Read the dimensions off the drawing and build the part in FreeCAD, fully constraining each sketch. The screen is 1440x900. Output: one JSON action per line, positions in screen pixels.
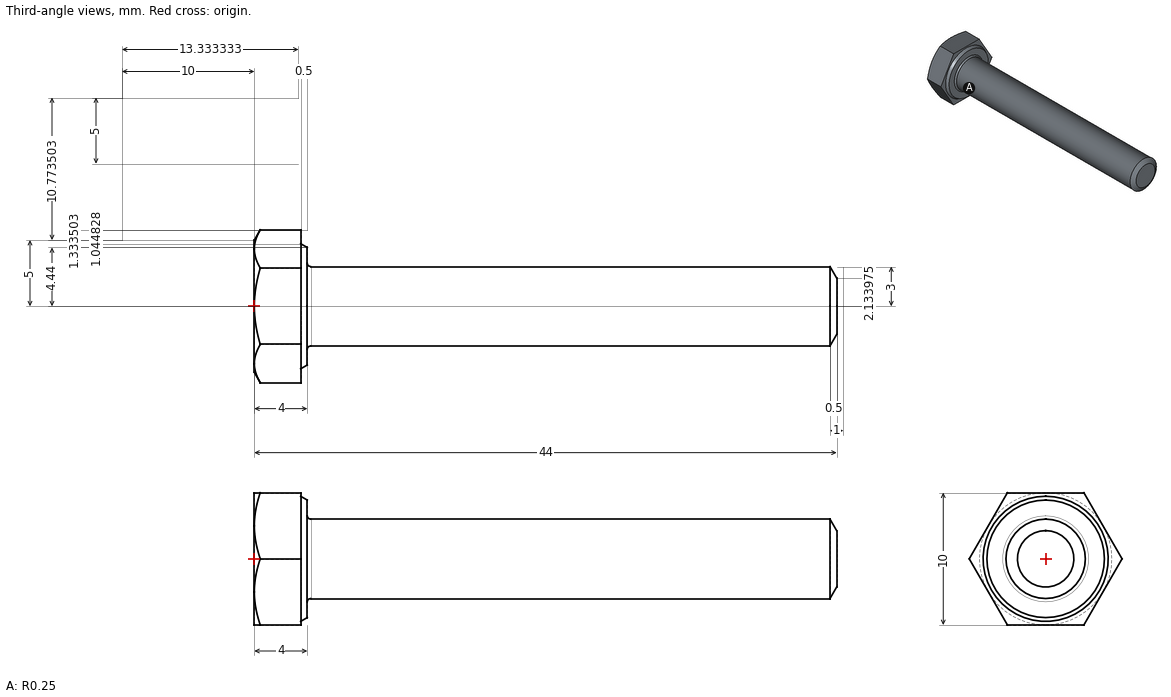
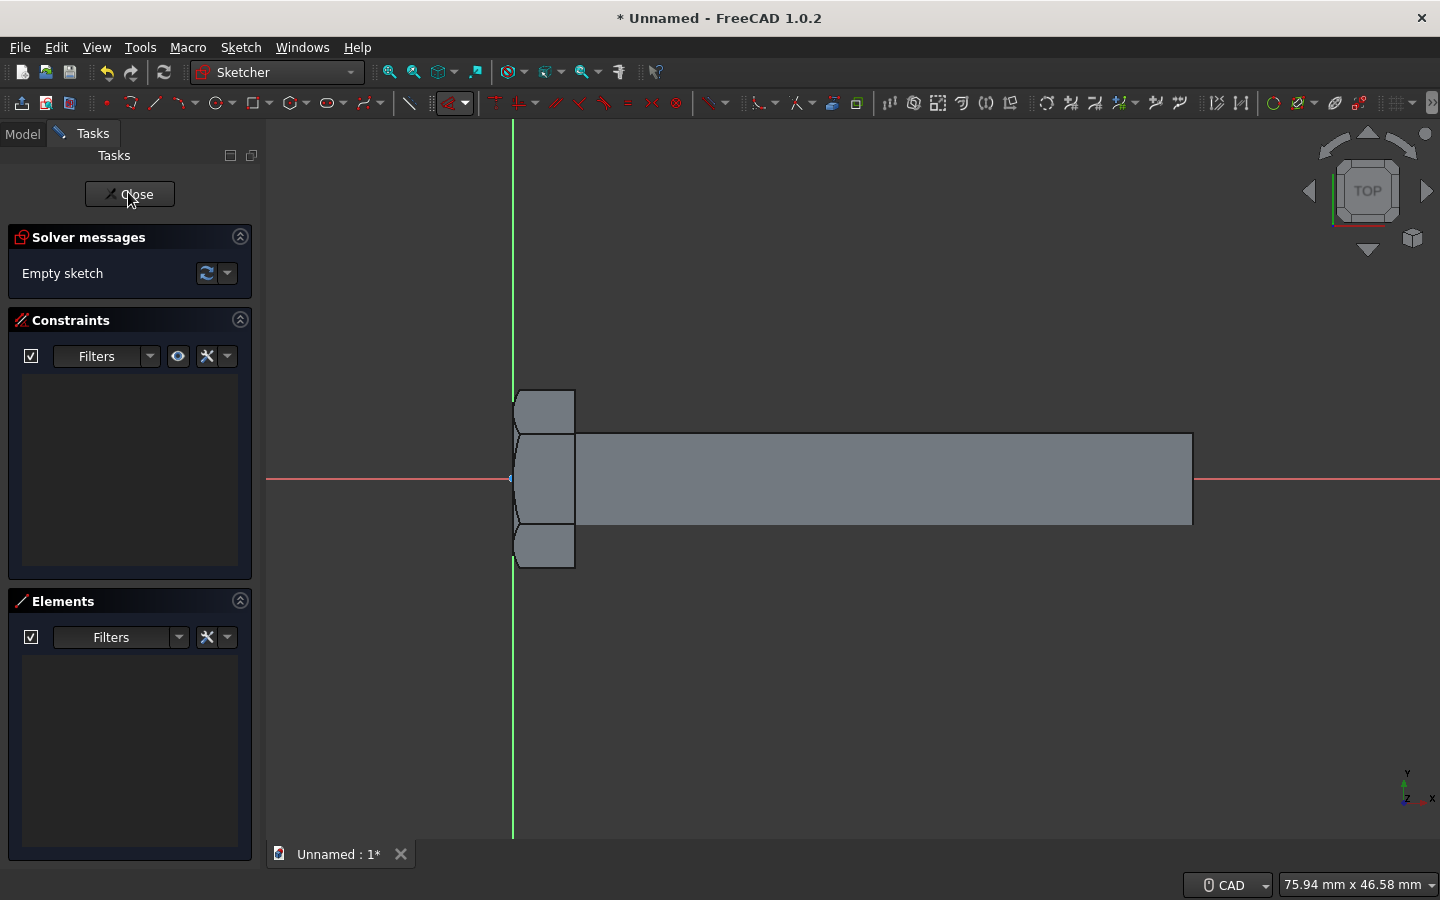
{"action": "left_click", "coordinate": [70, 104]}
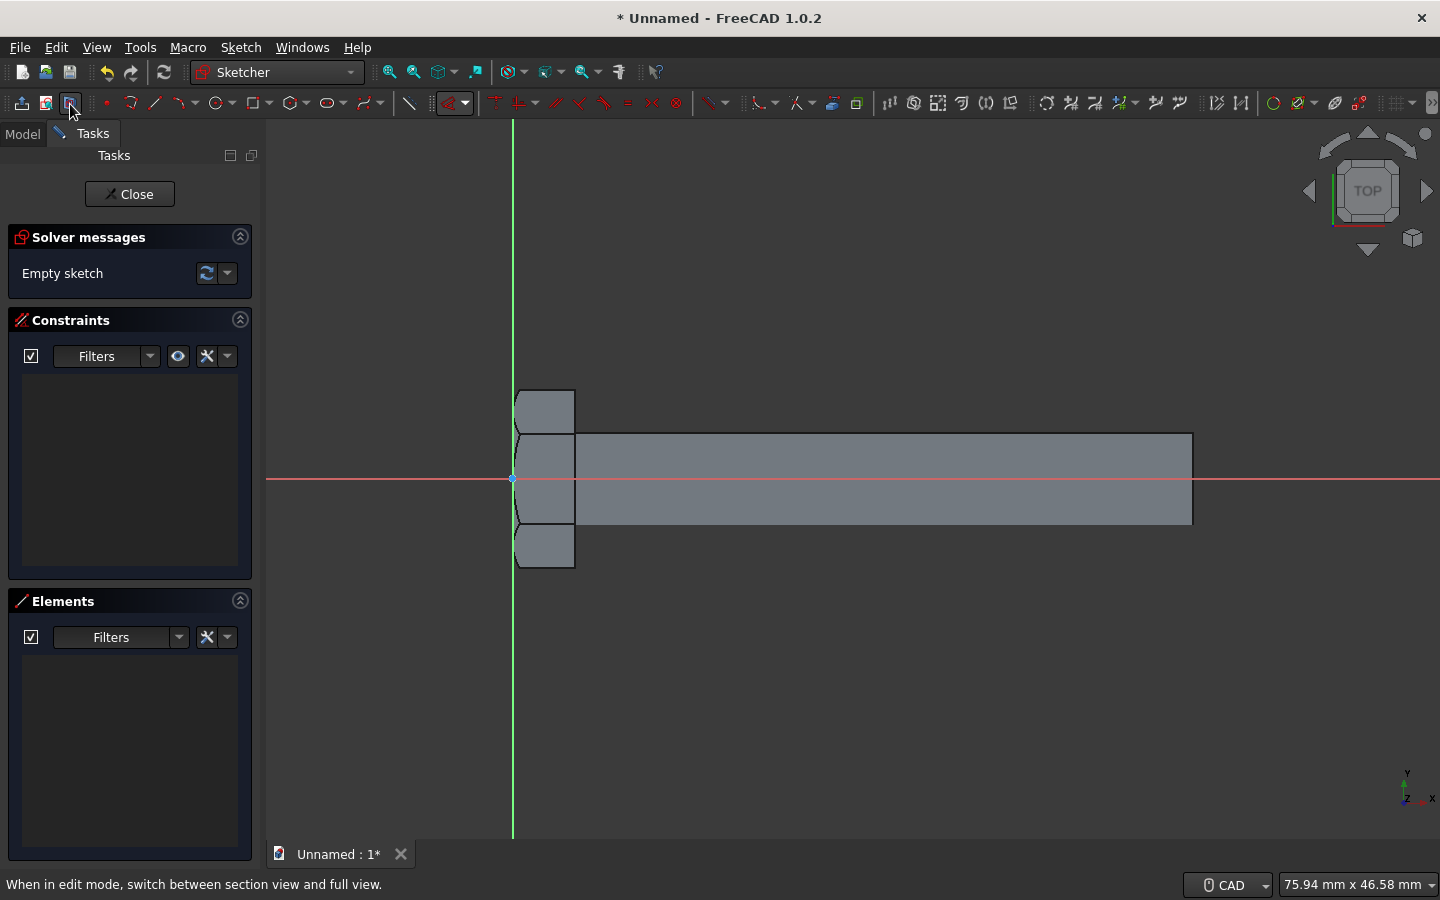
{"action": "scroll", "coordinate": [560, 396], "scroll_direction": "up", "scroll_amount": 15}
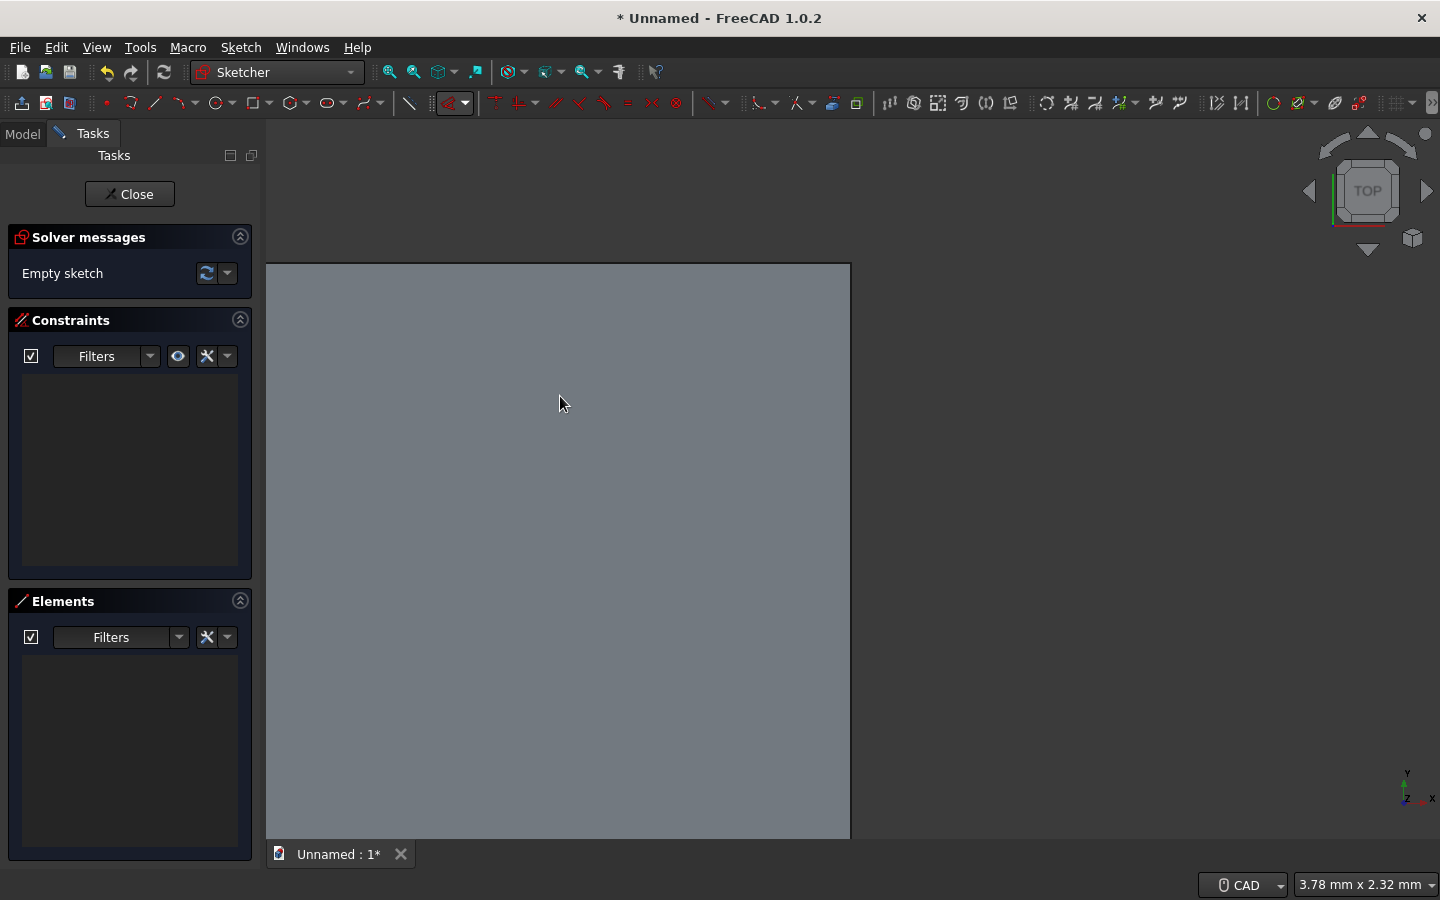
{"action": "left_click", "coordinate": [132, 104]}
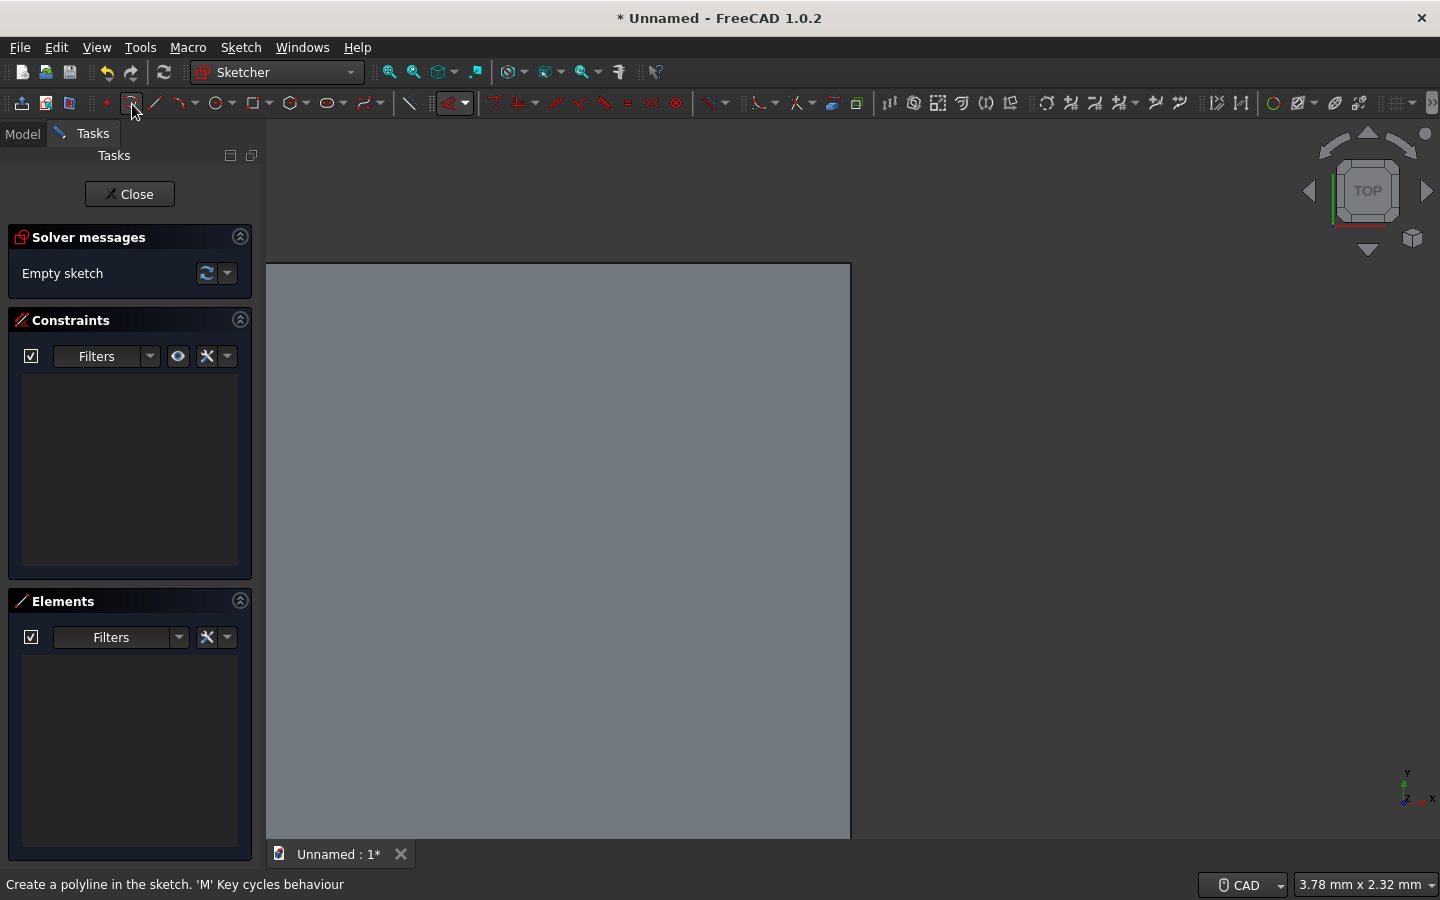
{"action": "left_click", "coordinate": [696, 588]}
{"action": "left_click", "coordinate": [851, 677]}
{"action": "left_click", "coordinate": [851, 263]}
{"action": "left_click", "coordinate": [696, 263]}
{"action": "left_click", "coordinate": [696, 589]}
{"action": "key", "text": "Escape"}
{"action": "key", "text": "Escape"}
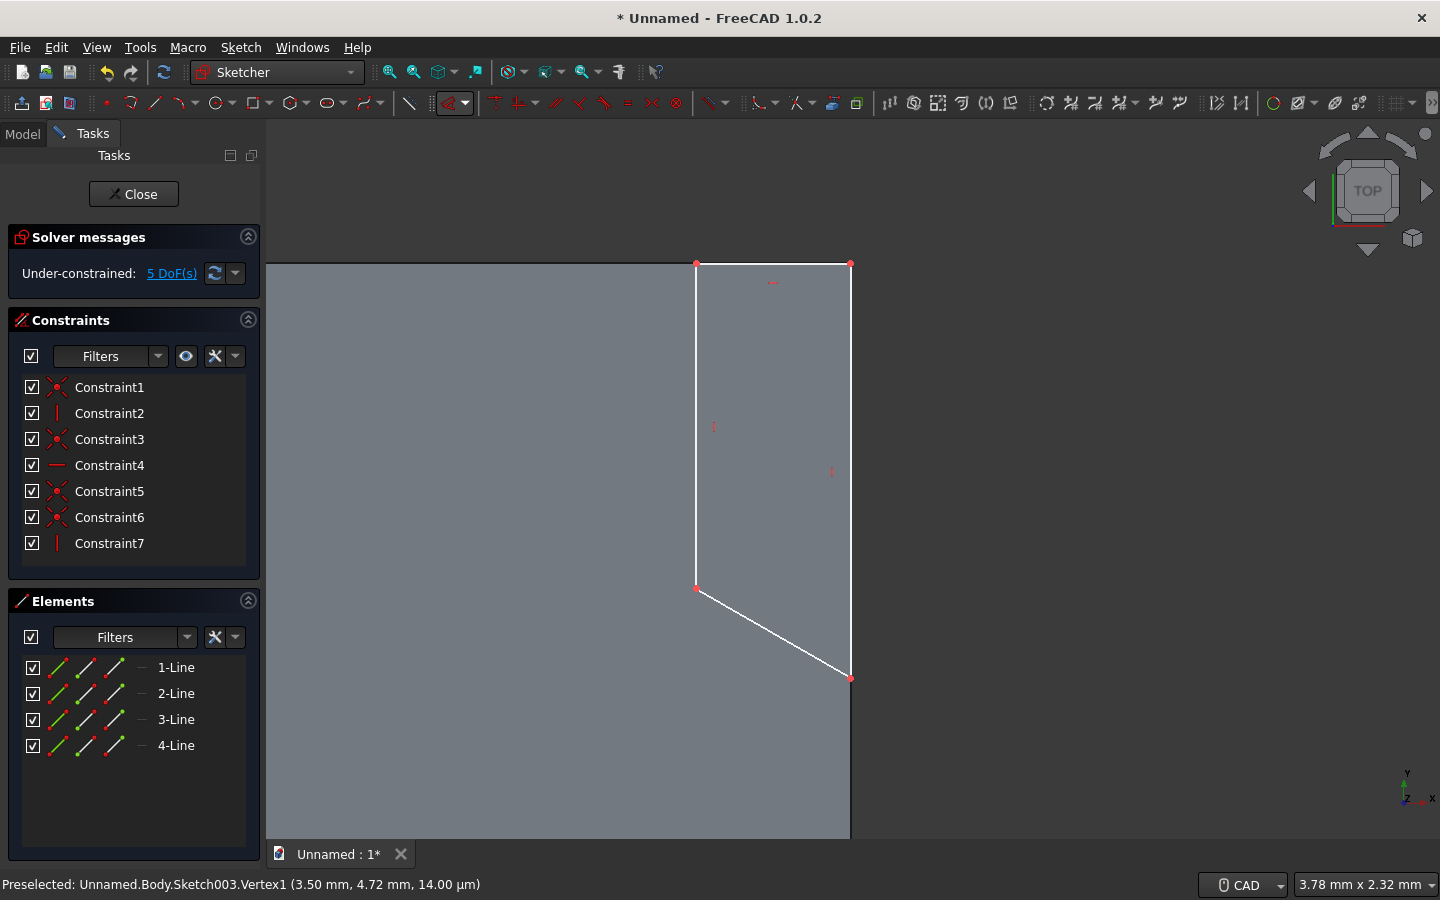
{"action": "left_click", "coordinate": [851, 678]}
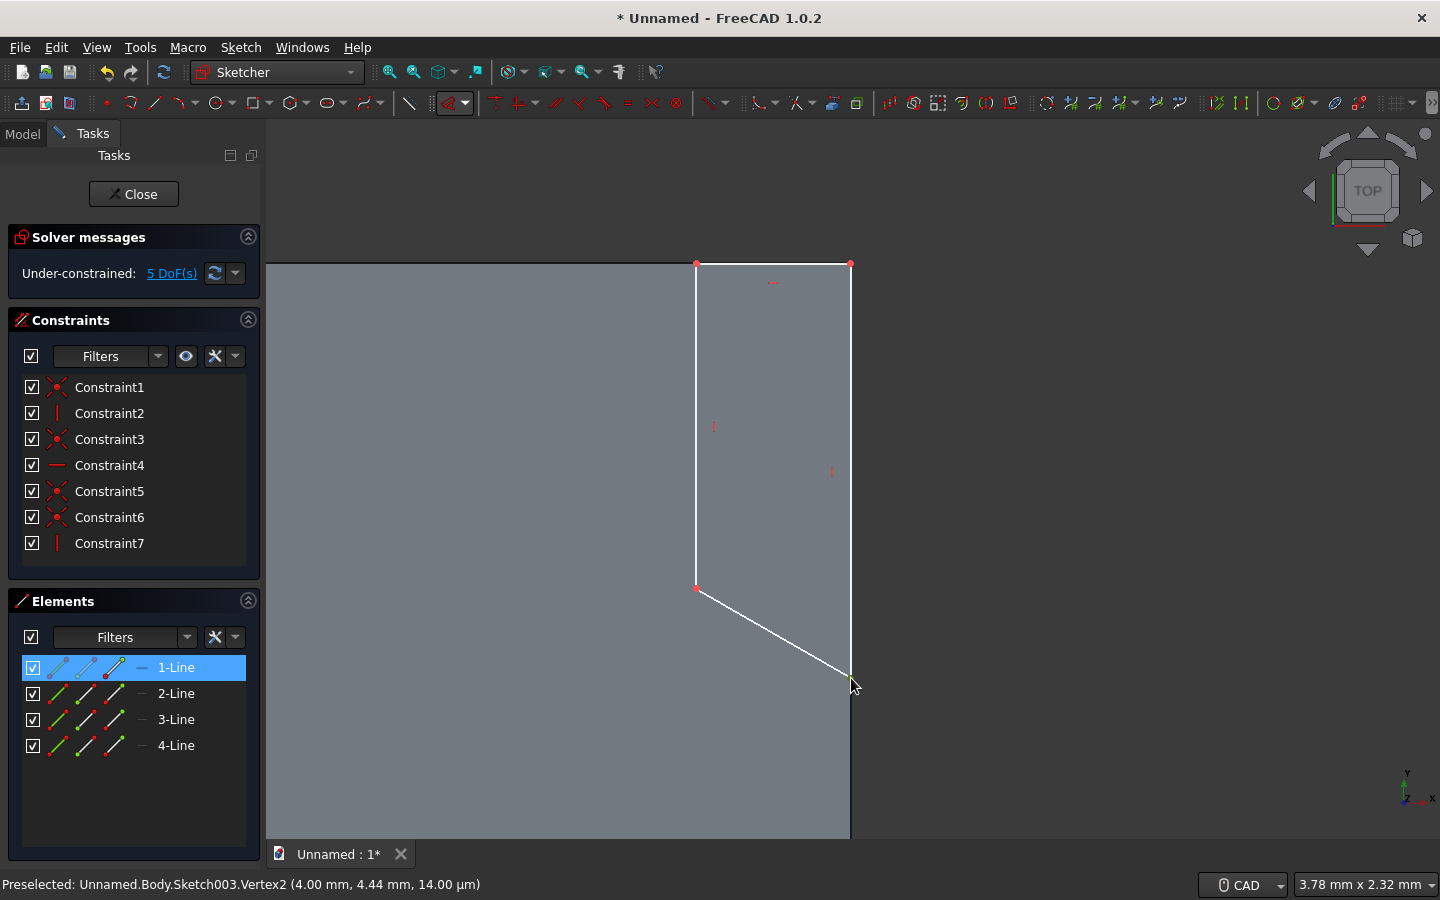
{"action": "left_click", "coordinate": [468, 104]}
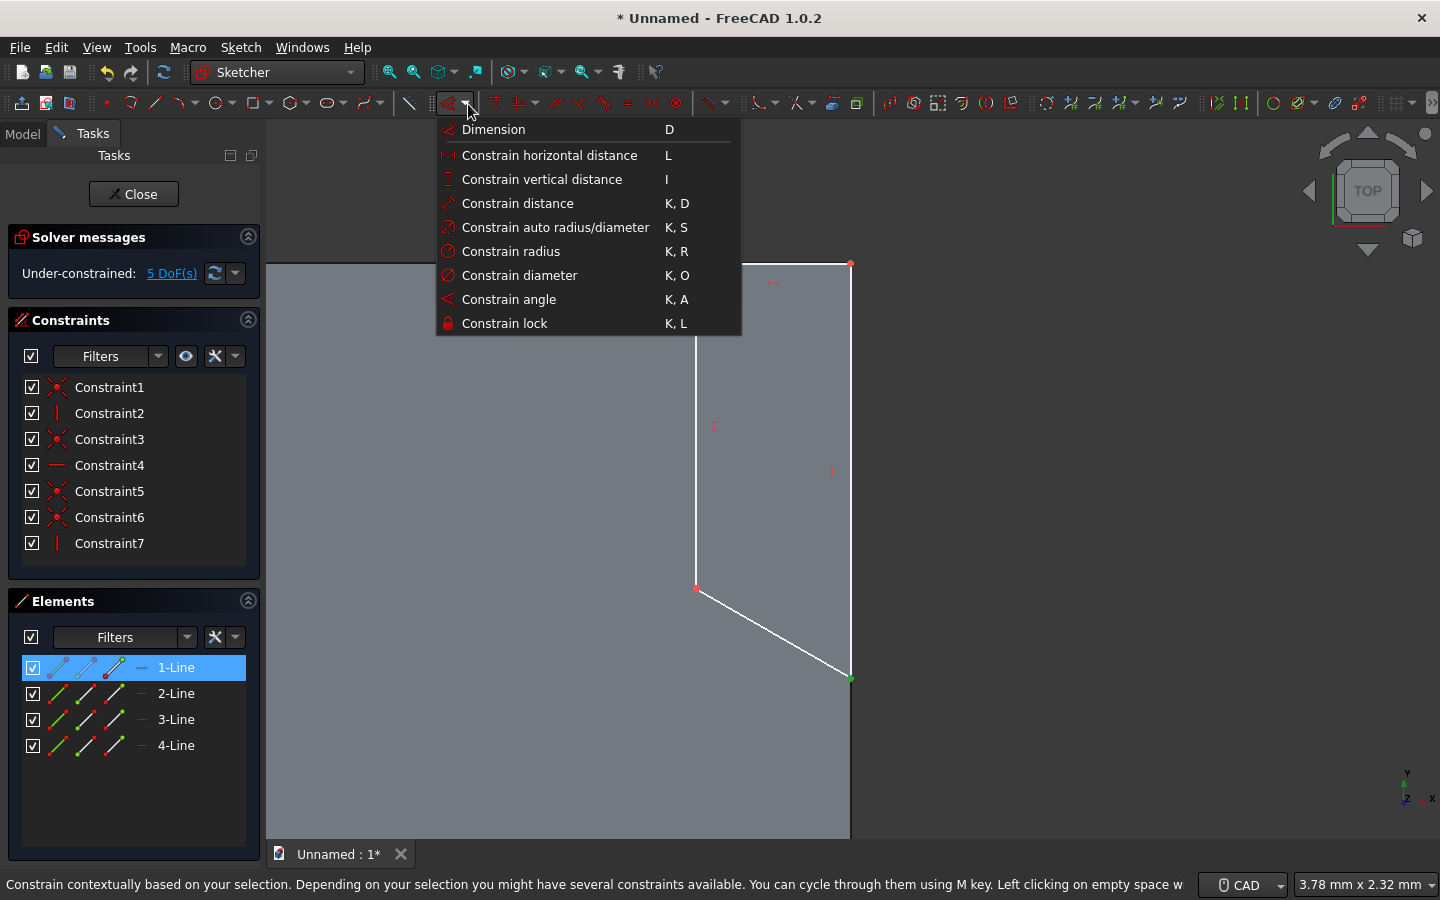
{"action": "left_click", "coordinate": [589, 155]}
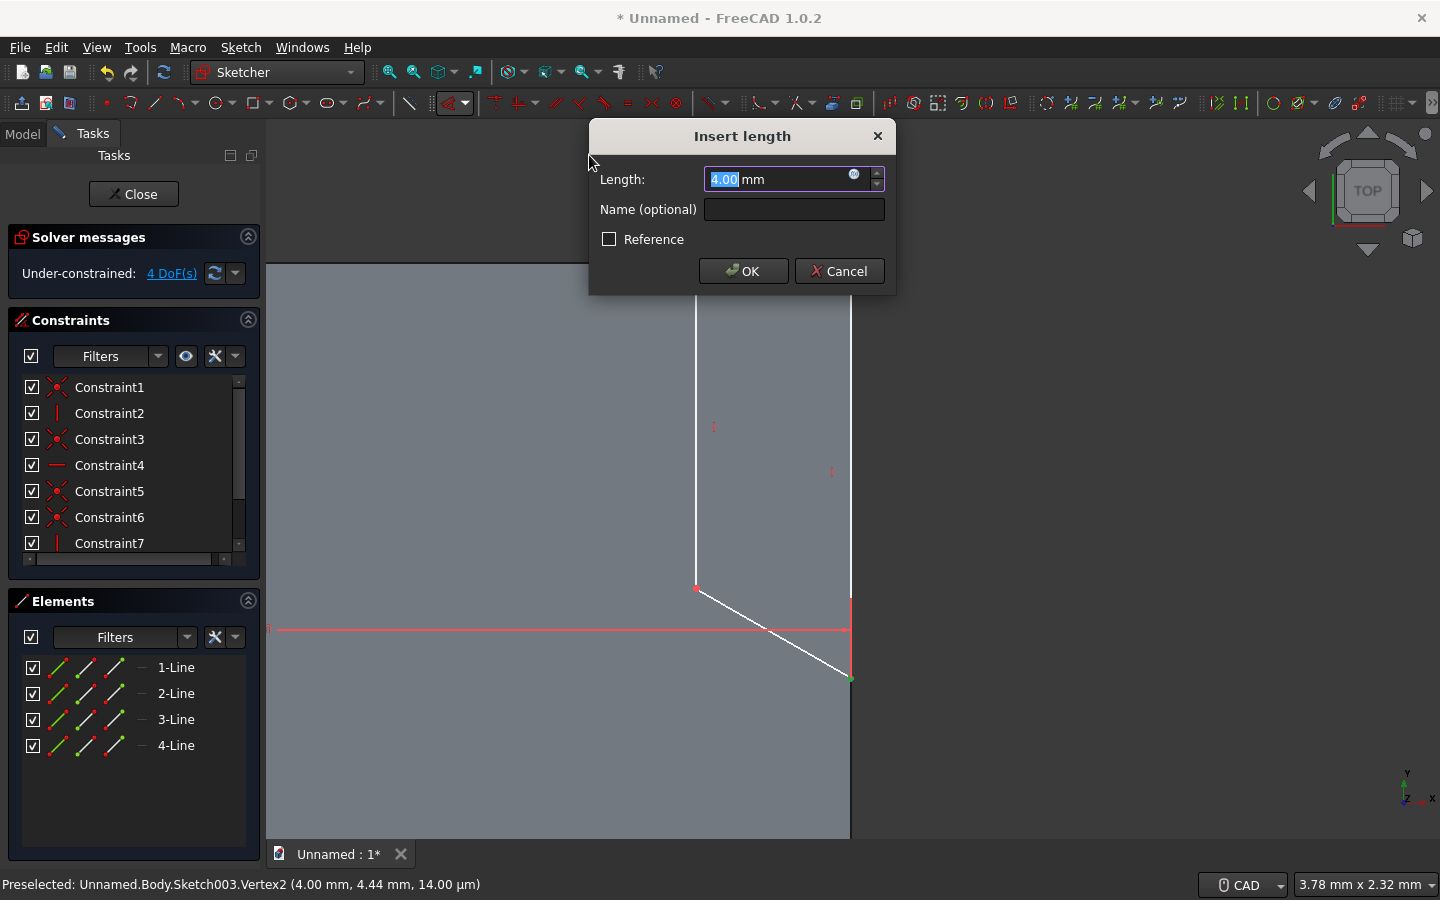
{"action": "type", "text": "4"}
{"action": "key", "text": "Return"}